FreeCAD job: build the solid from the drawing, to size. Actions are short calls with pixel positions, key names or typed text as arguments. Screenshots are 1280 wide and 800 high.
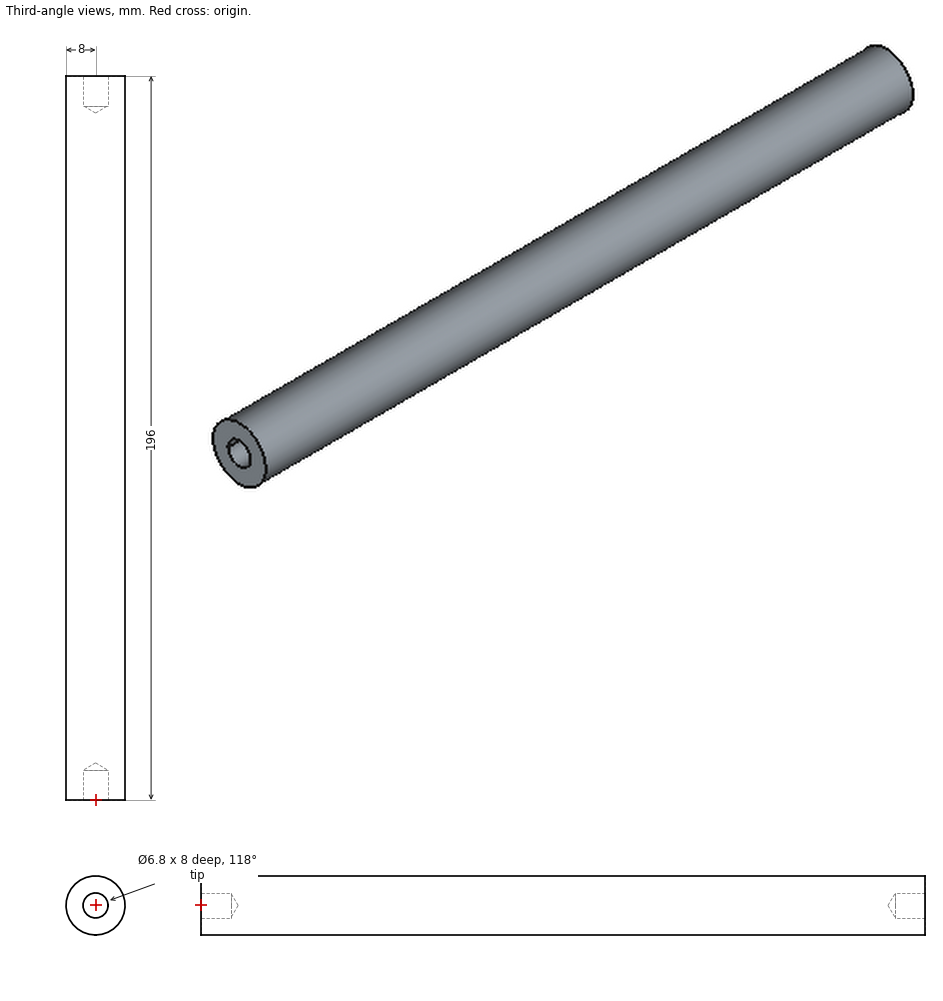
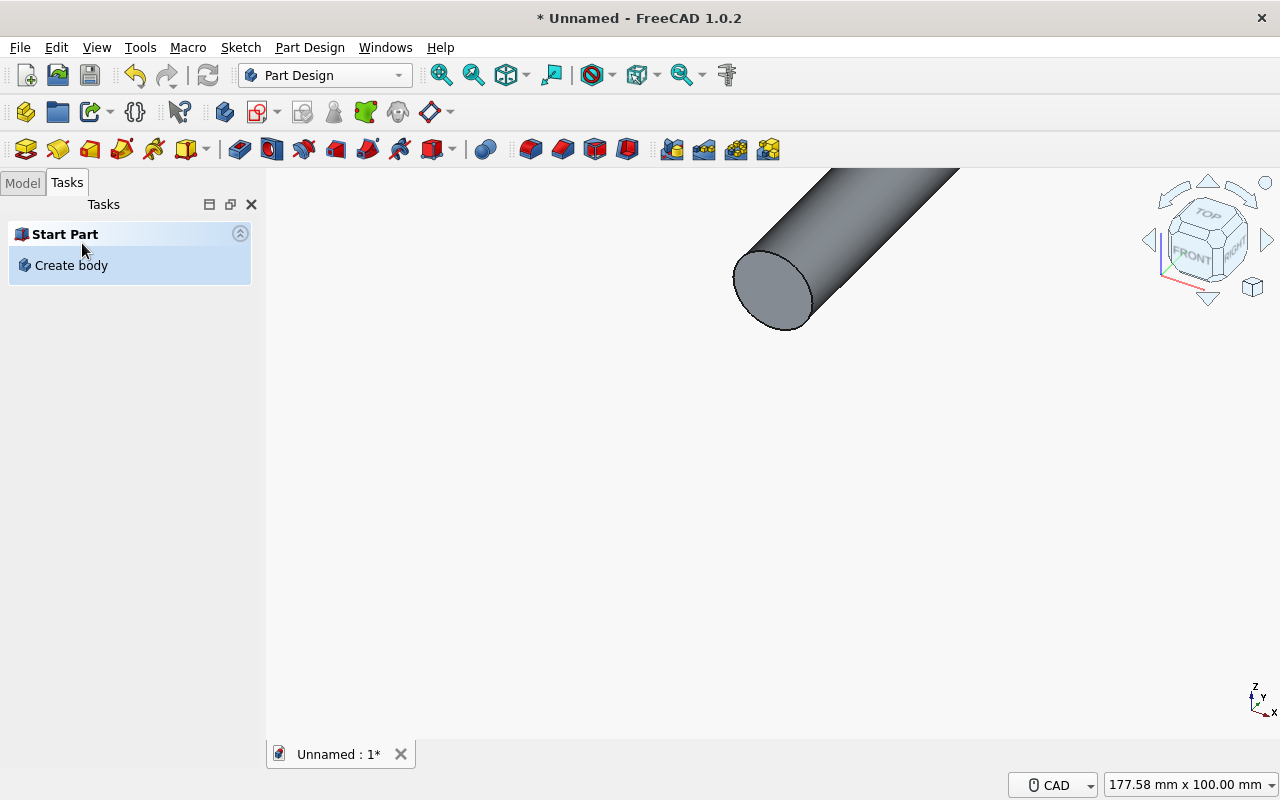
click(442, 76)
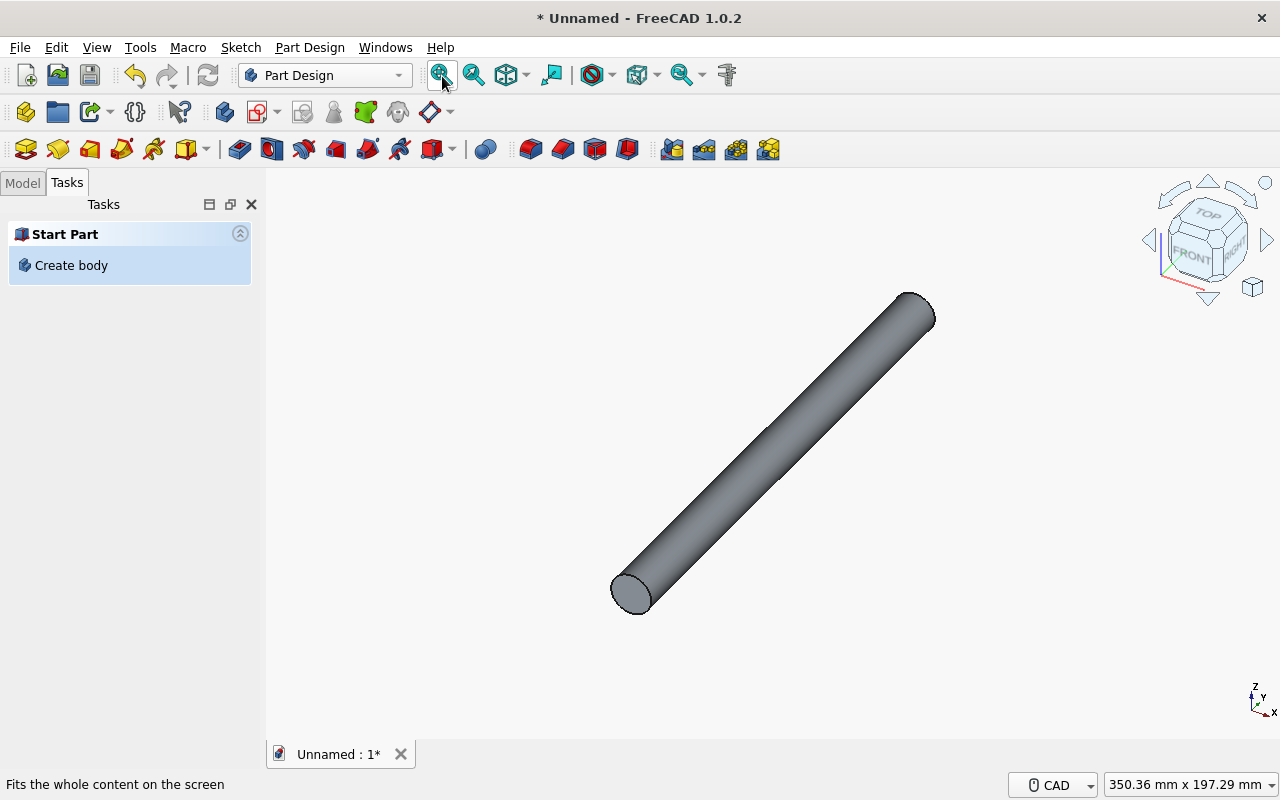
click(631, 593)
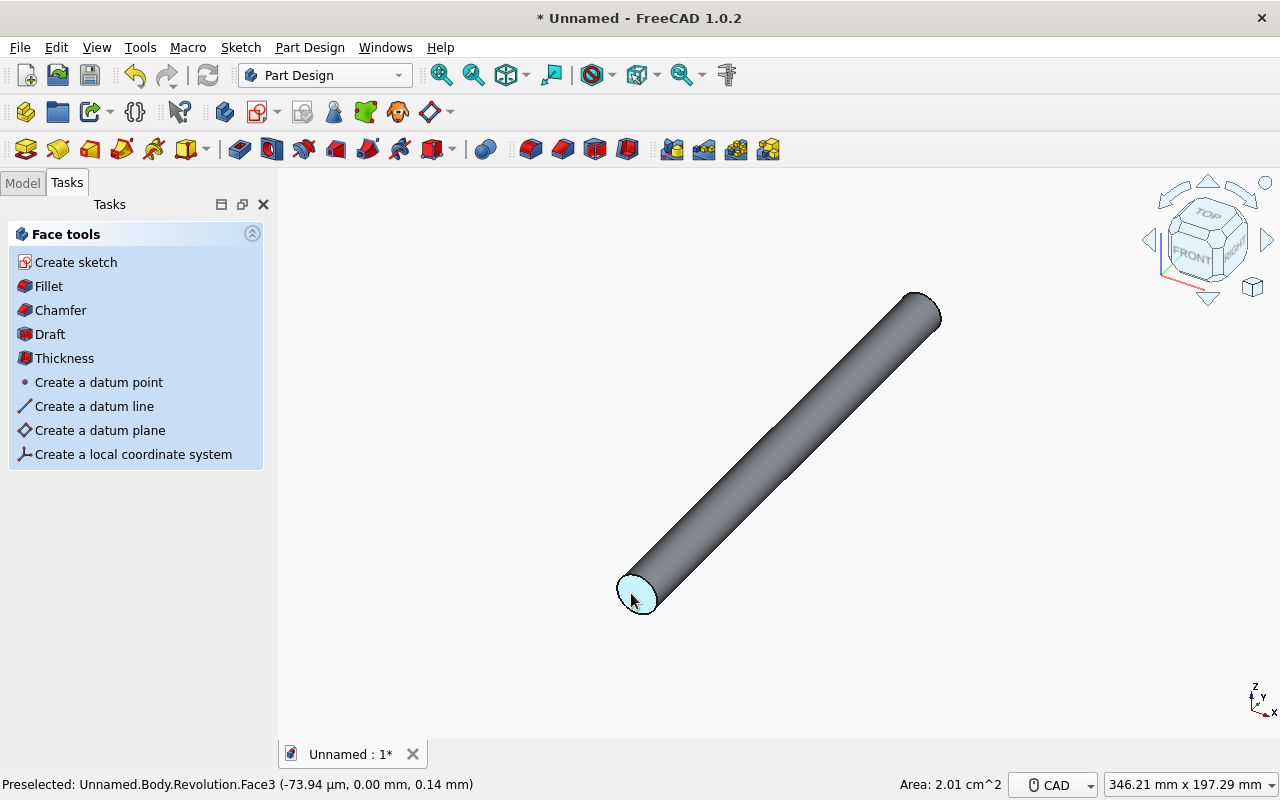
click(258, 112)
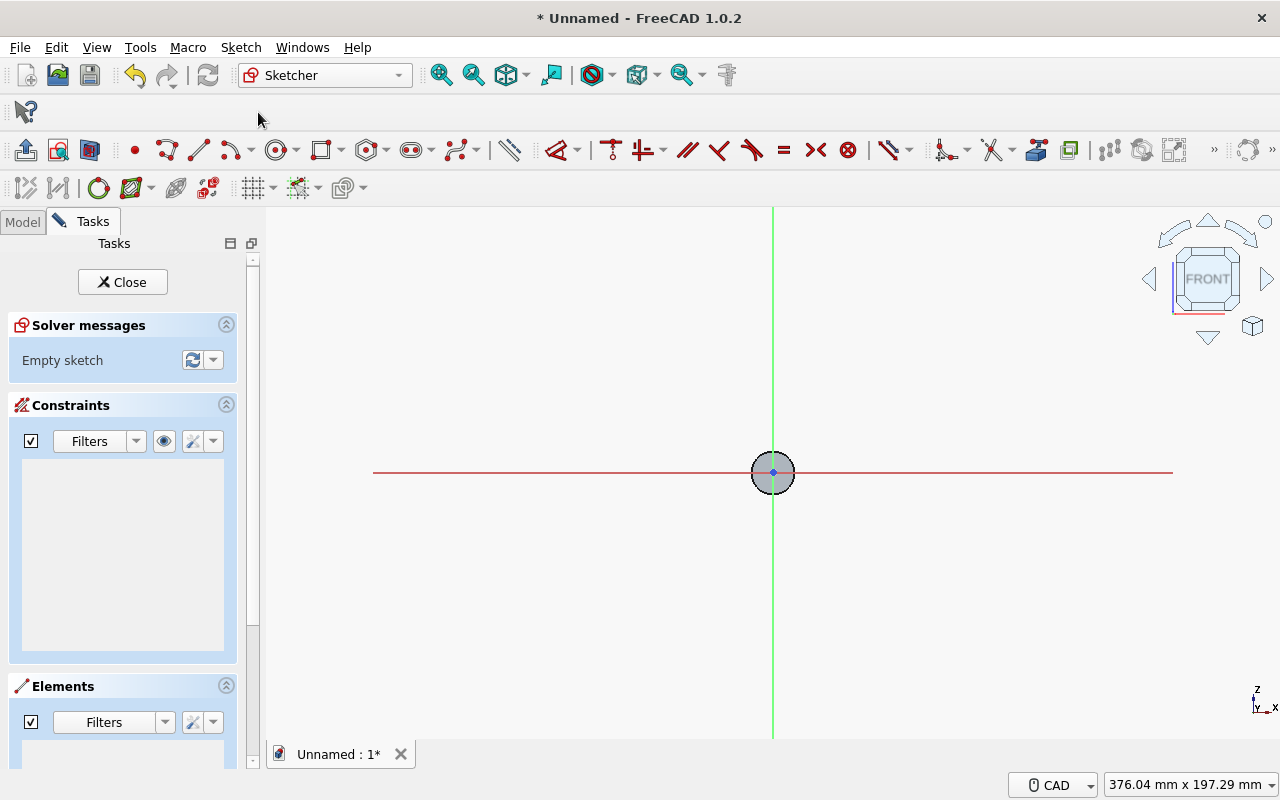
scroll(777, 473, up, 15)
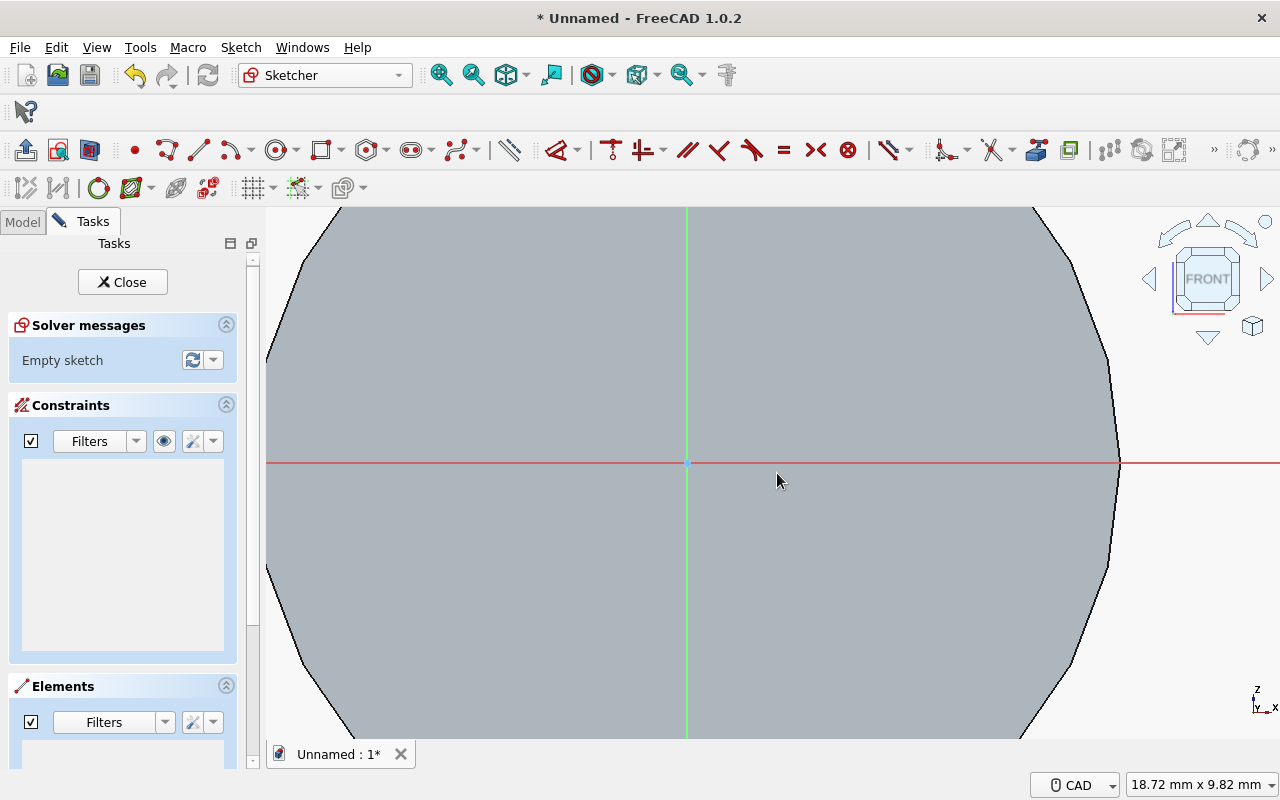
click(276, 150)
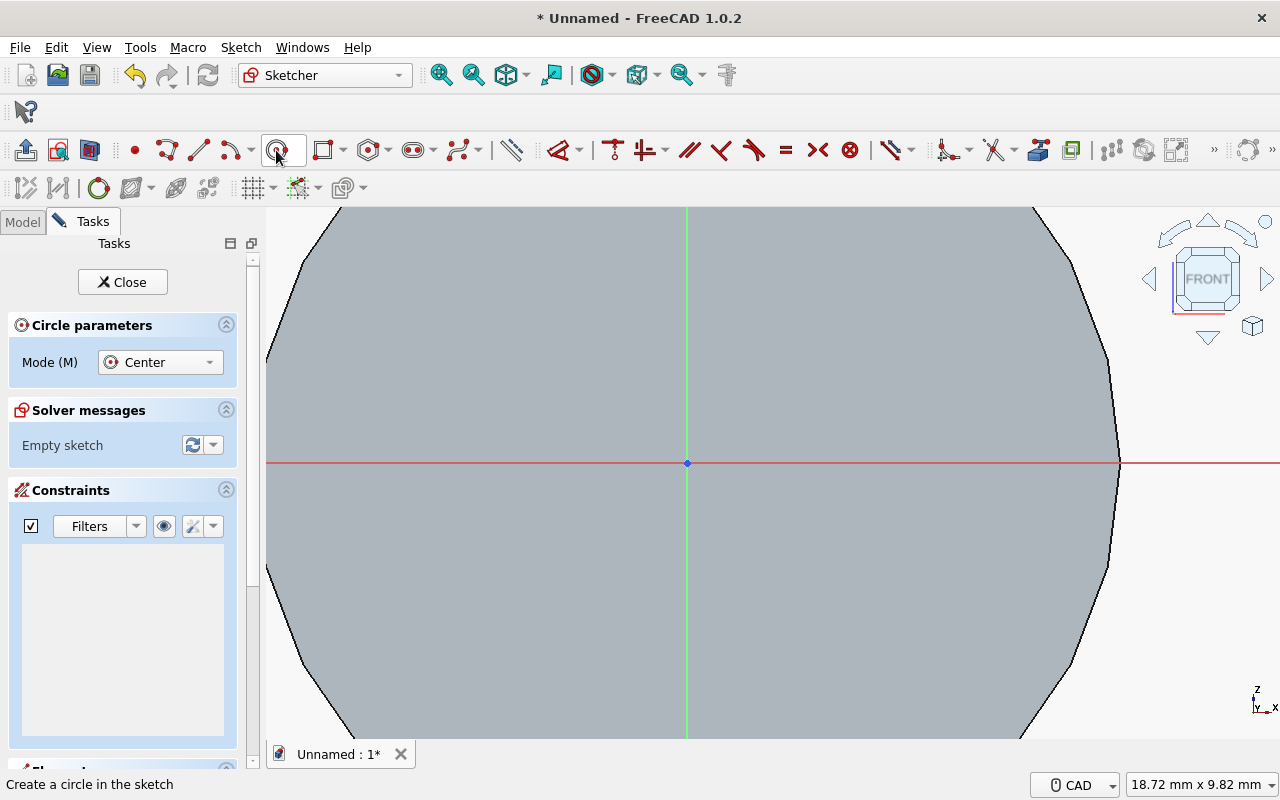
click(687, 463)
move(817, 333)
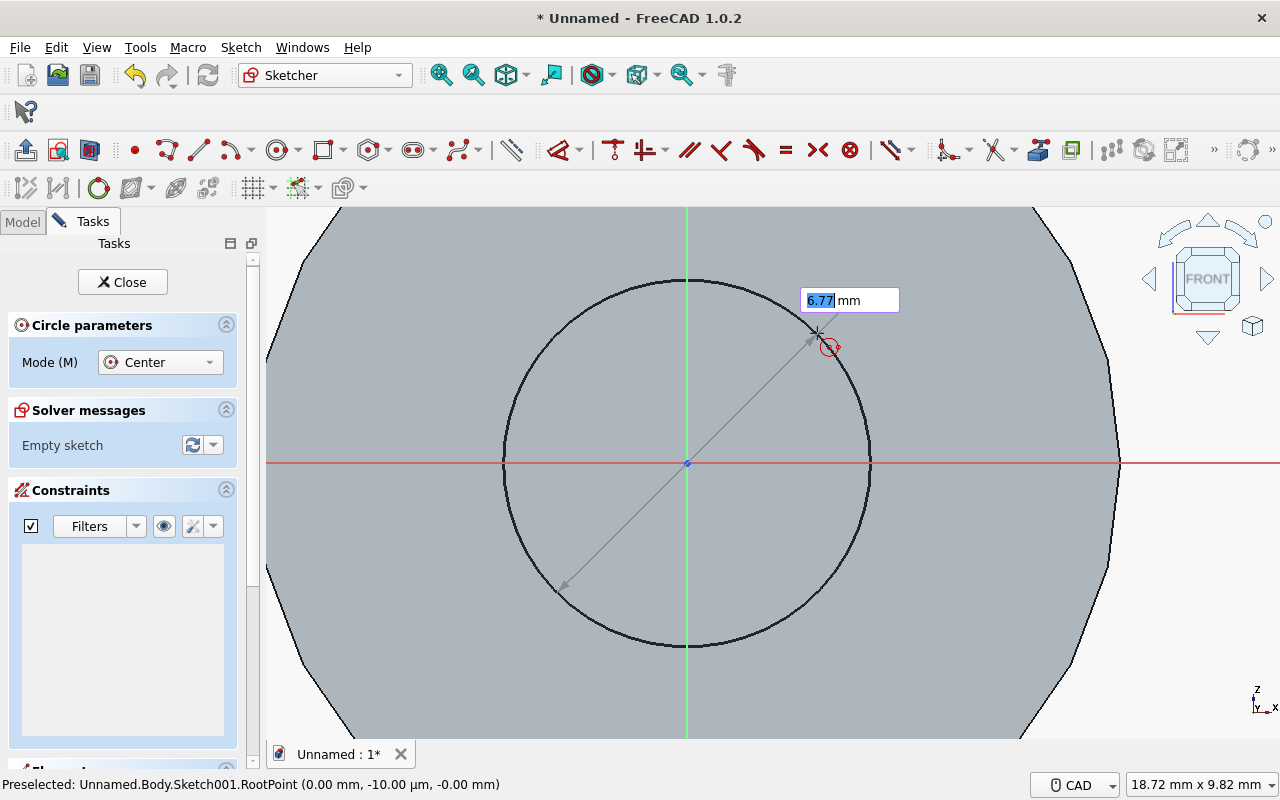
text(6.8)
key(Return)
key(Escape)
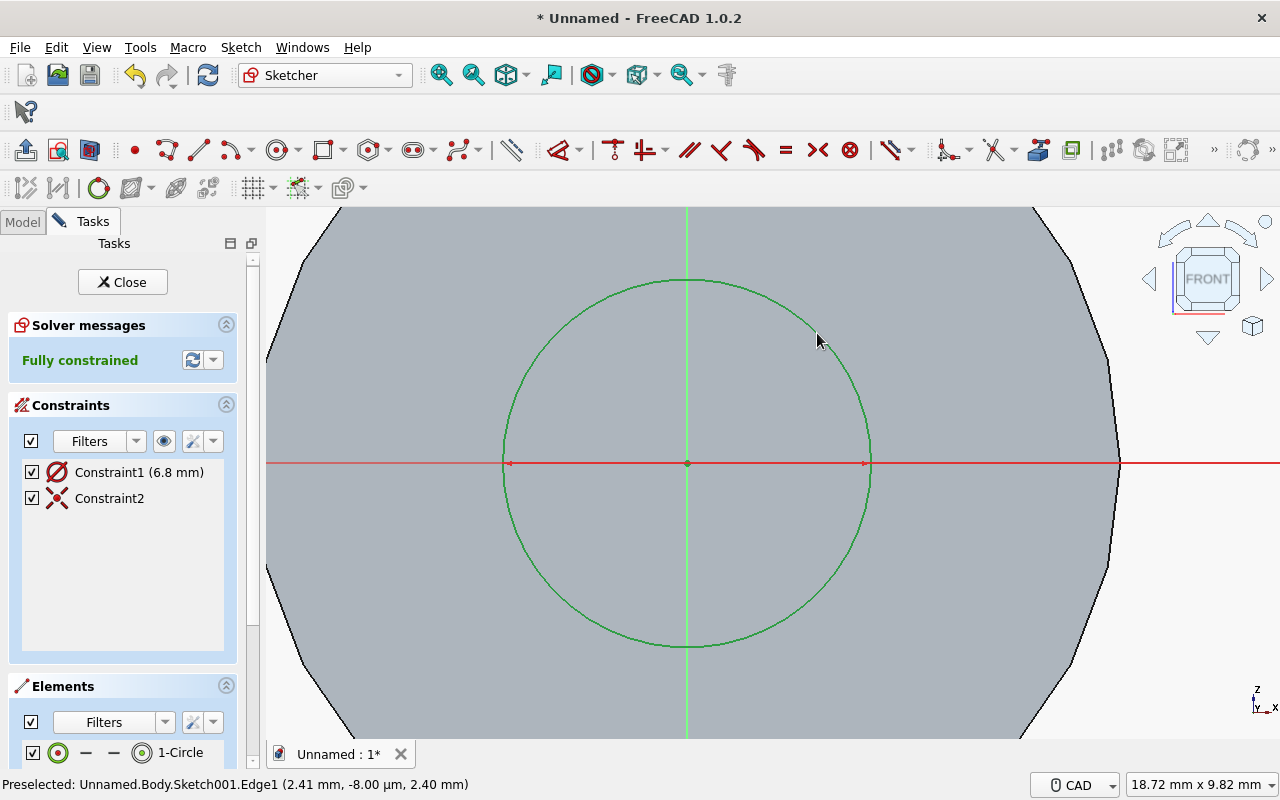
click(123, 282)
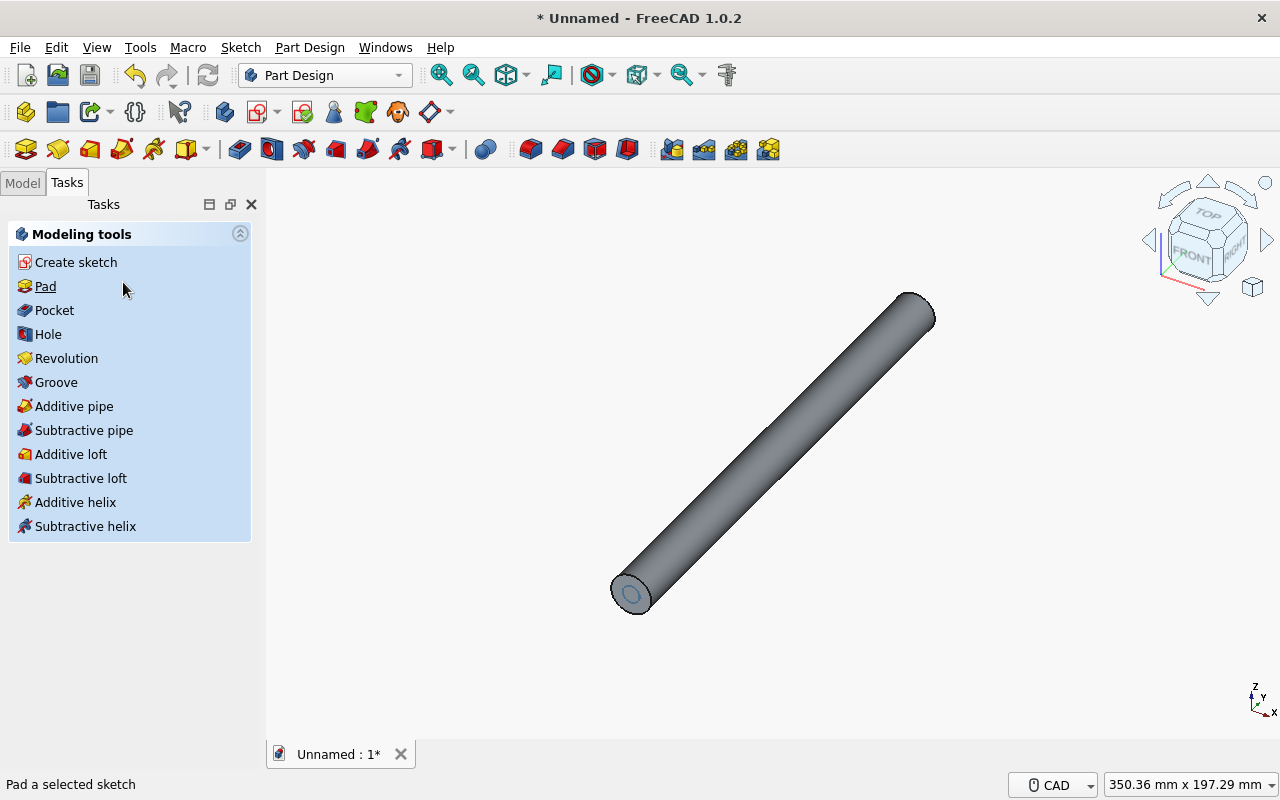
click(272, 150)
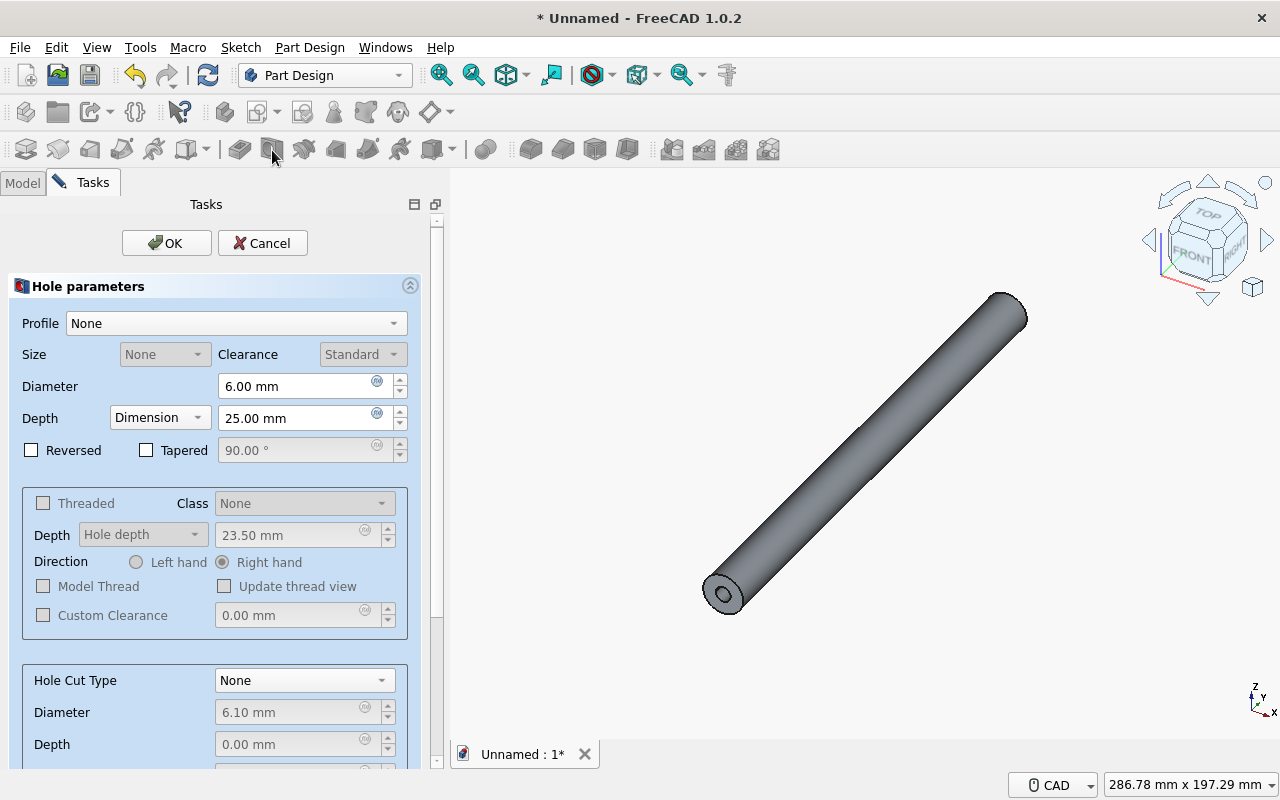
triple_click(305, 386)